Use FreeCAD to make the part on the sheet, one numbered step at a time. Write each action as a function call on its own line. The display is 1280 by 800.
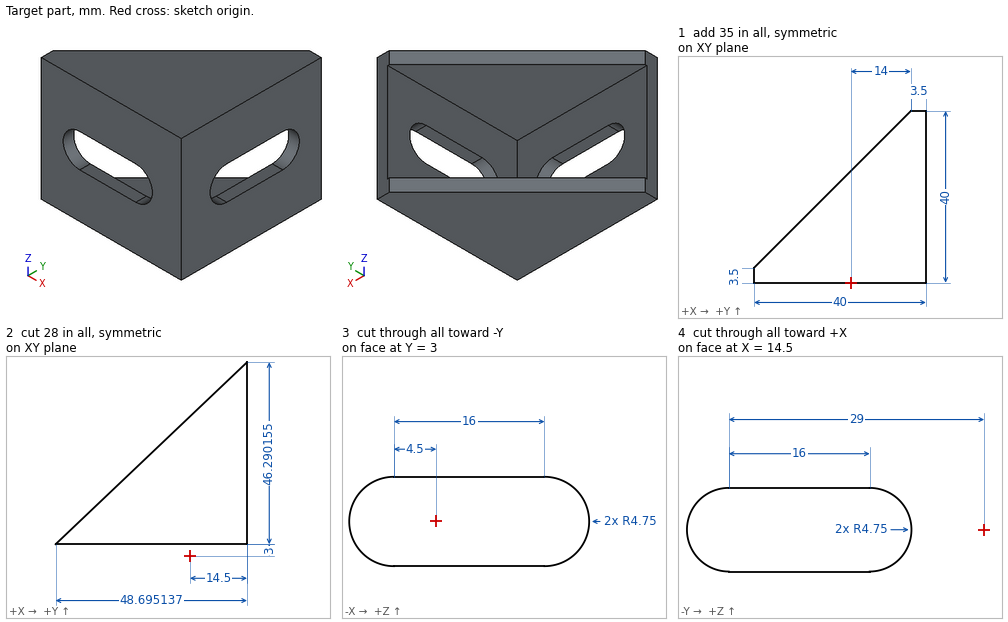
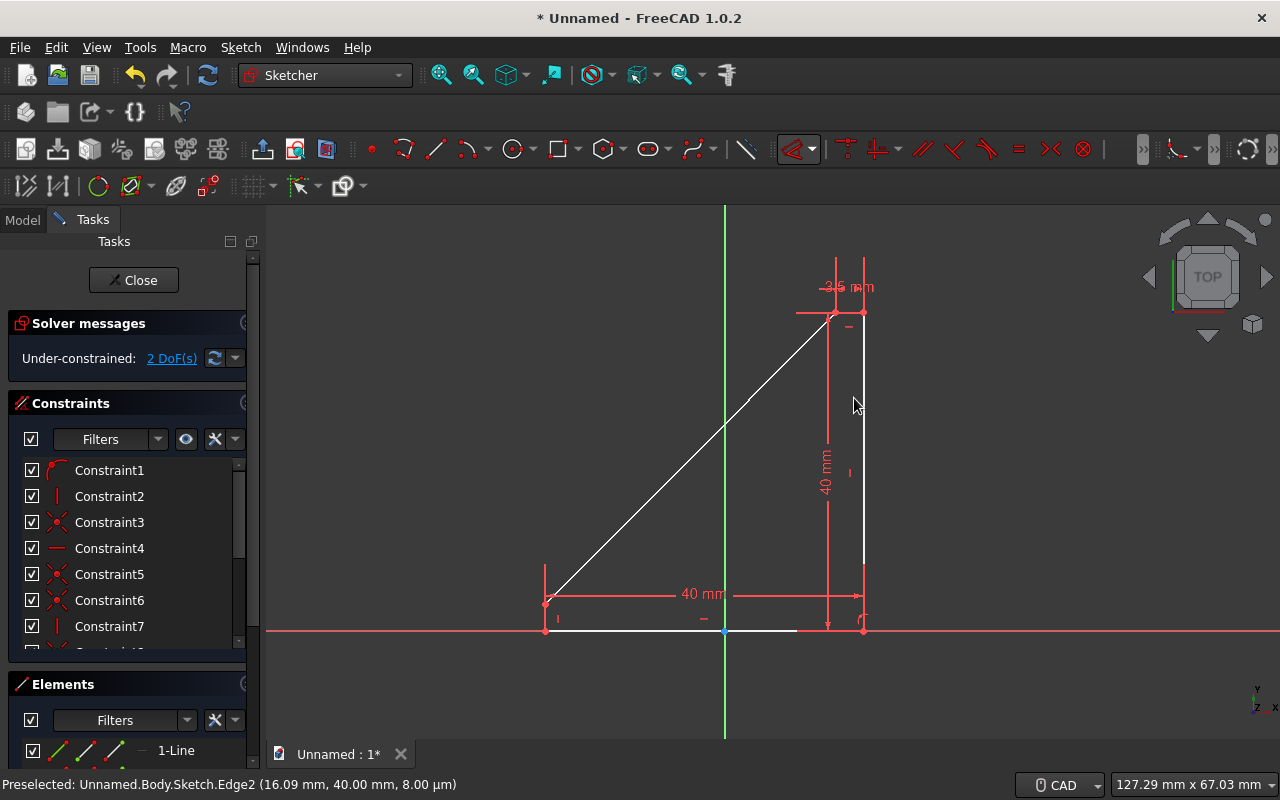
scroll(545, 613, up, 3)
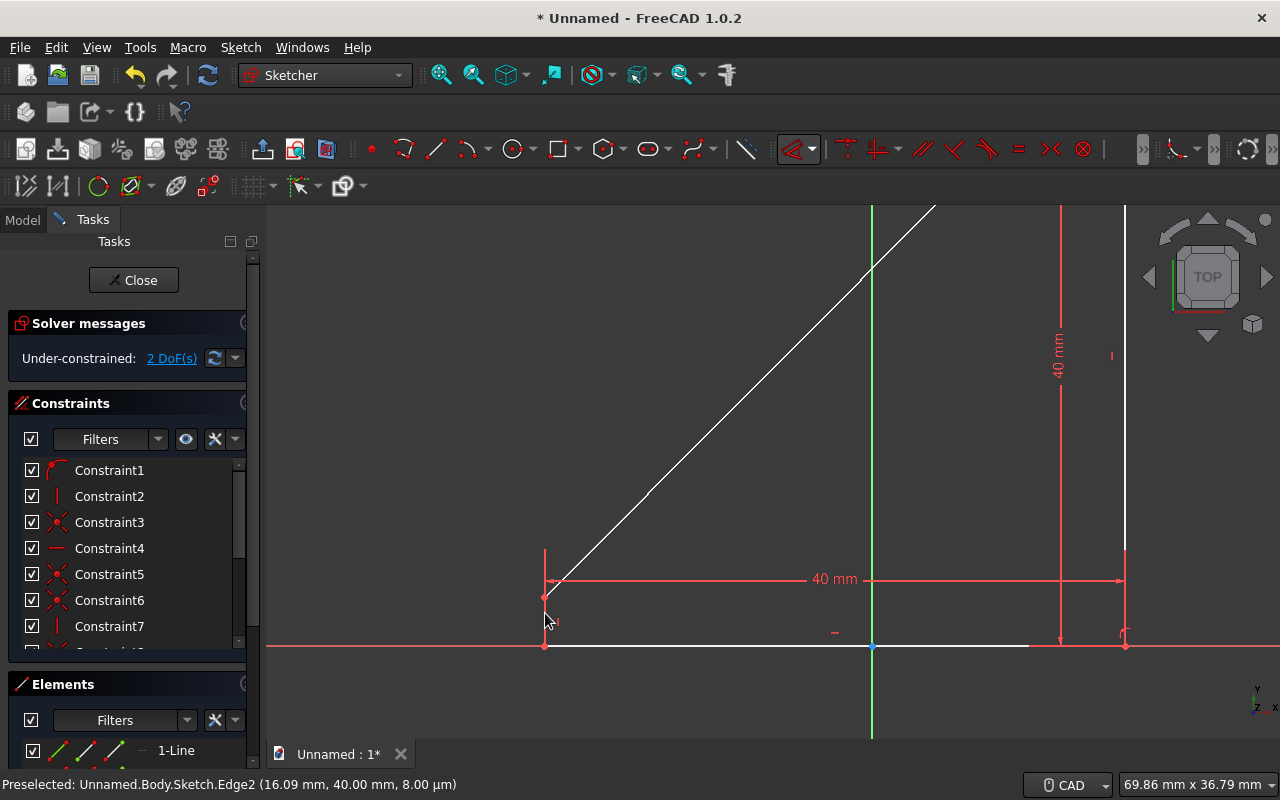
click(545, 612)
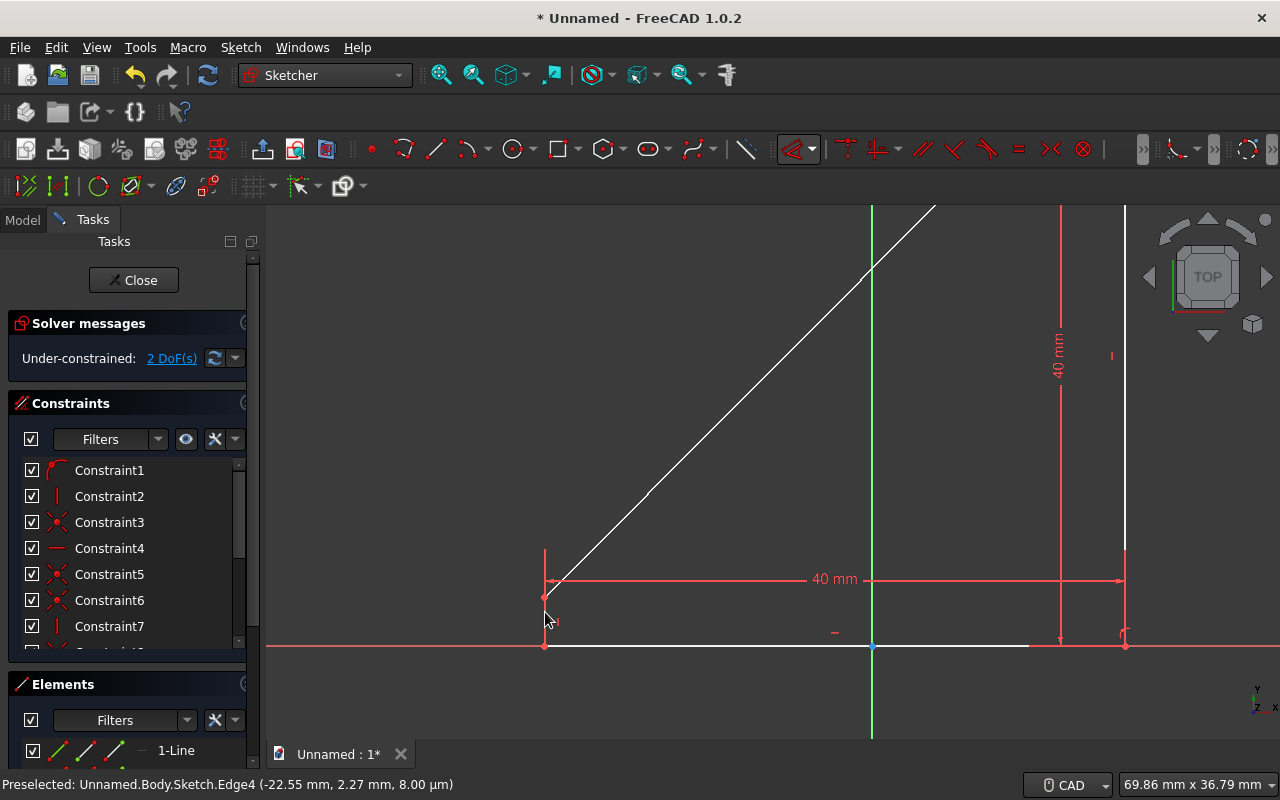
key(i)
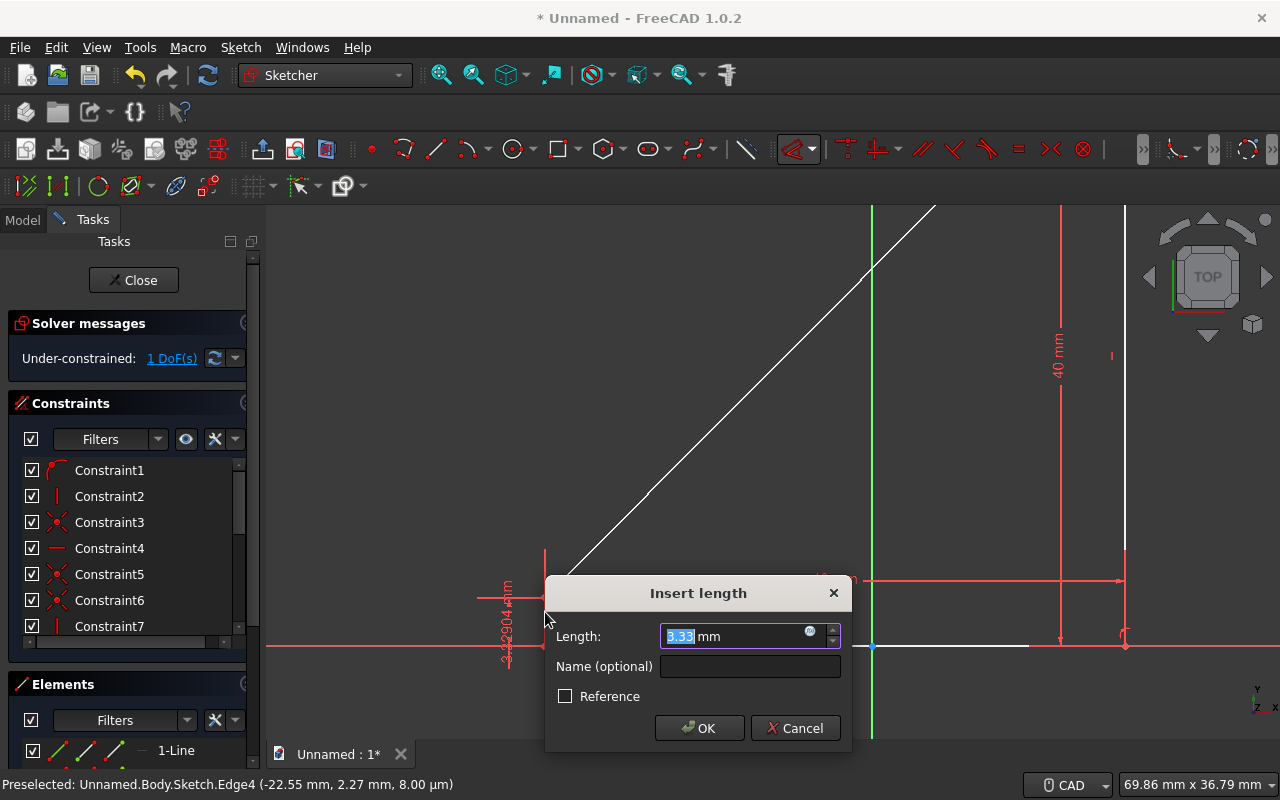
text(3.5)
key(Return)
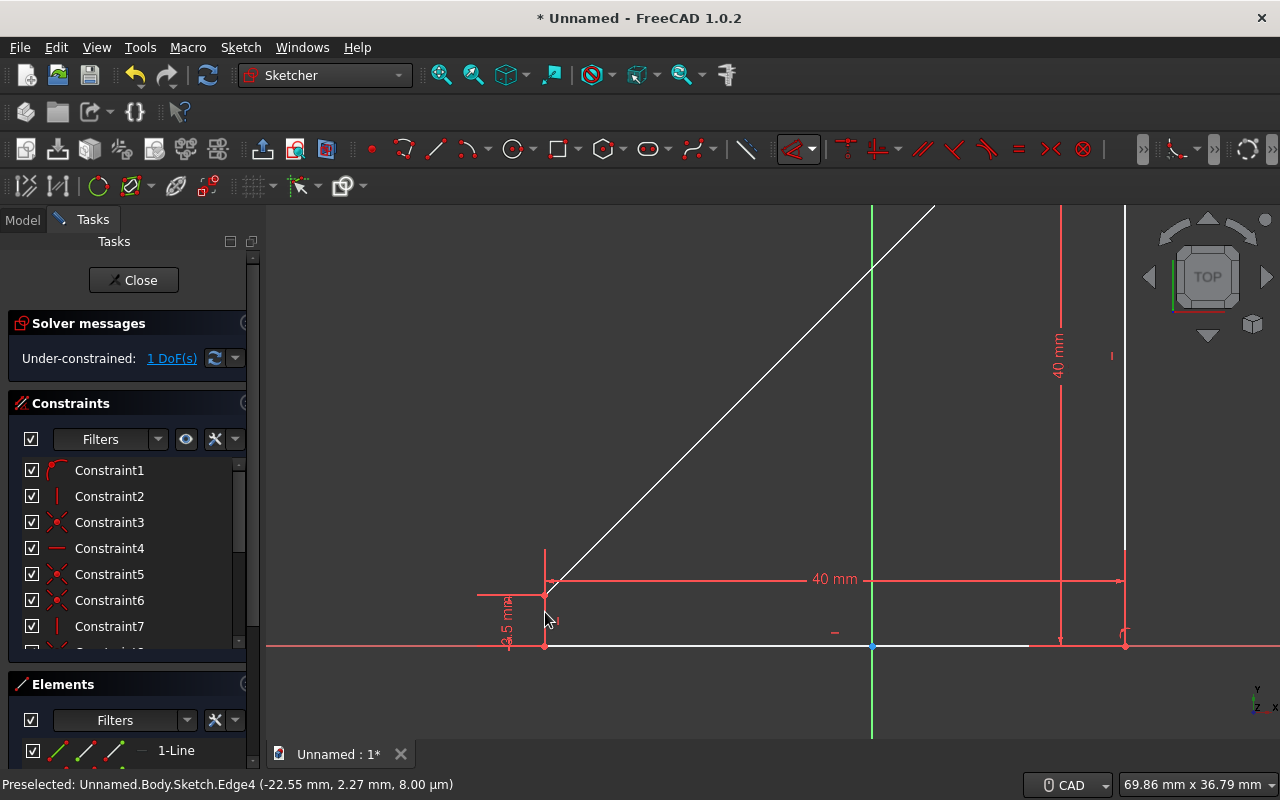
scroll(545, 613, down, 3)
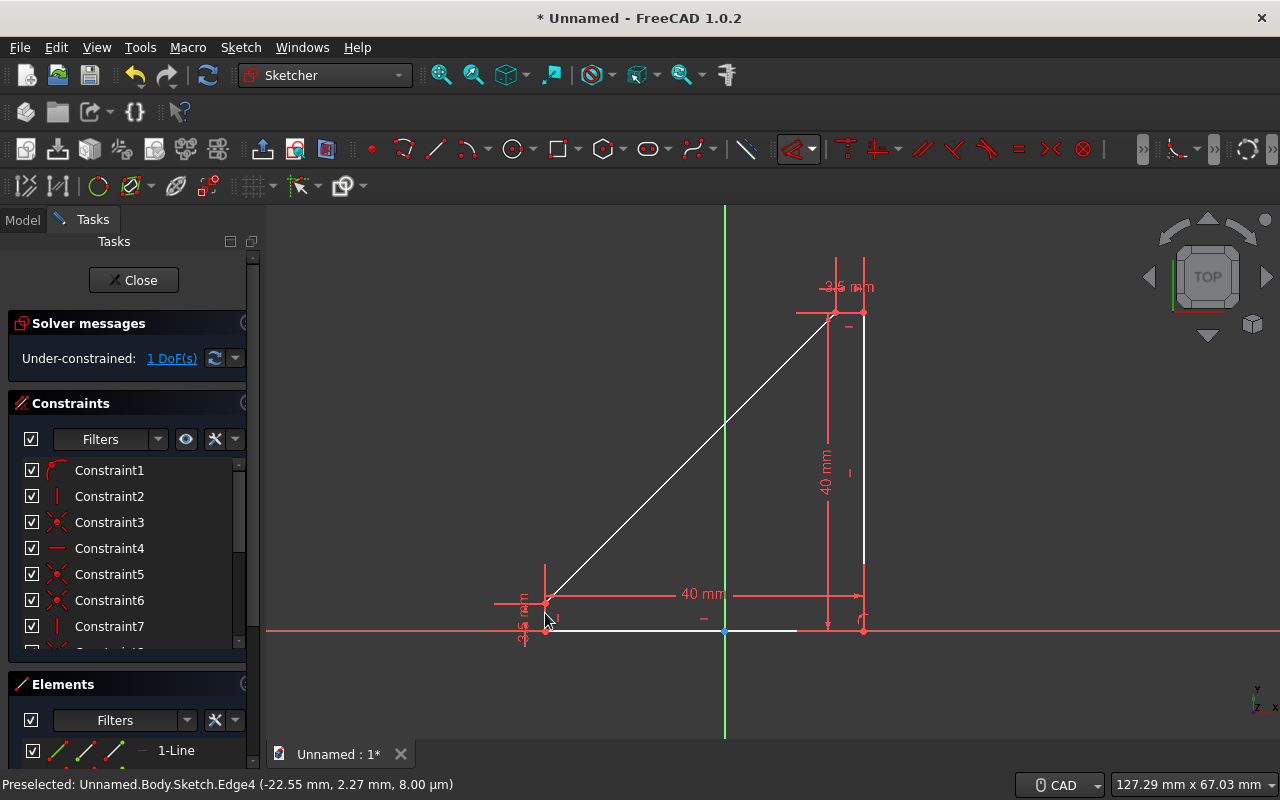
click(836, 313)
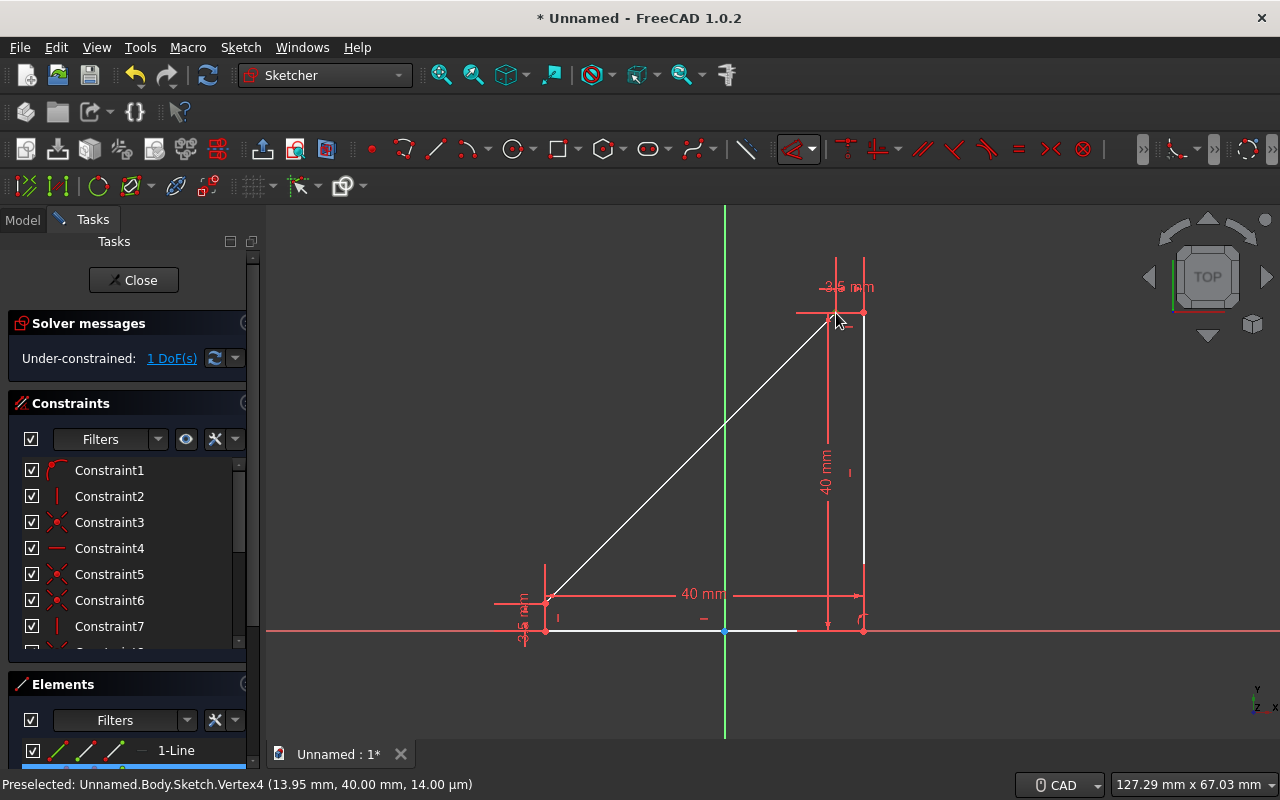
key(l)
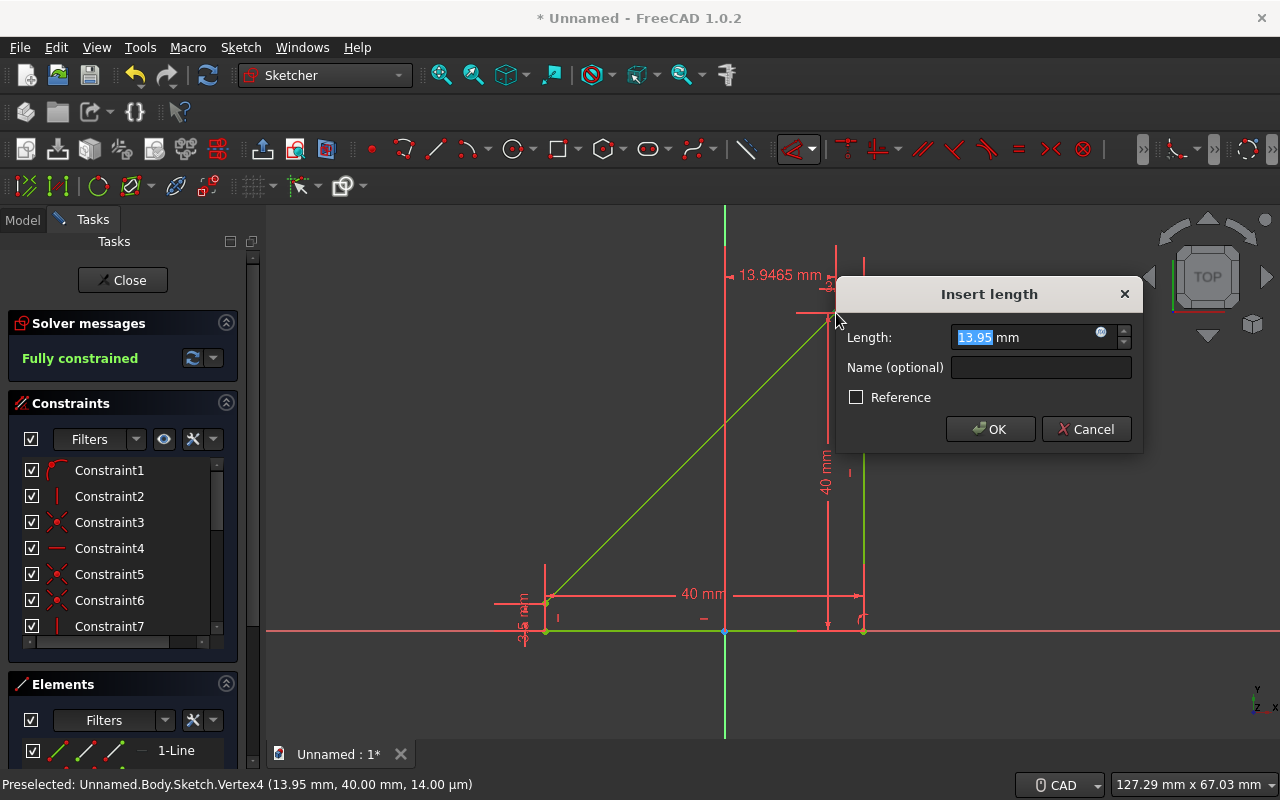
text(14)
key(Return)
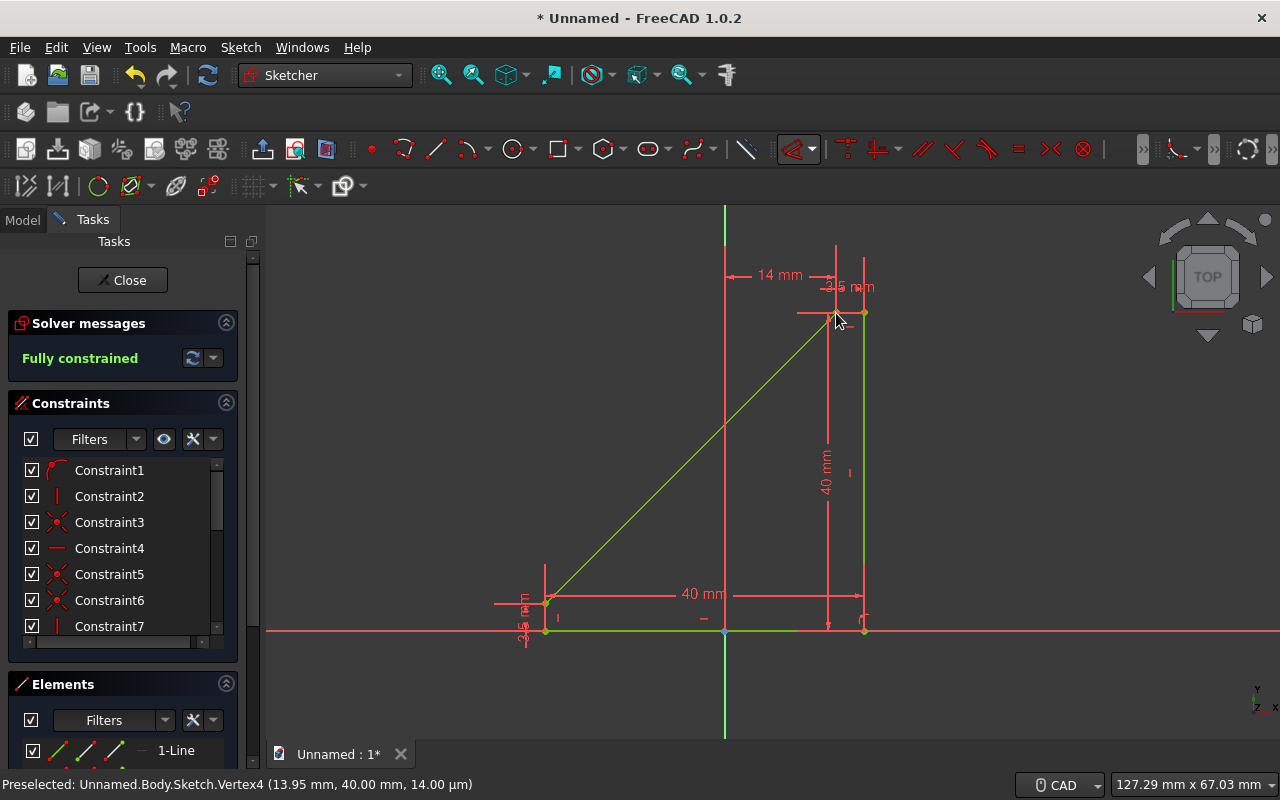
click(123, 280)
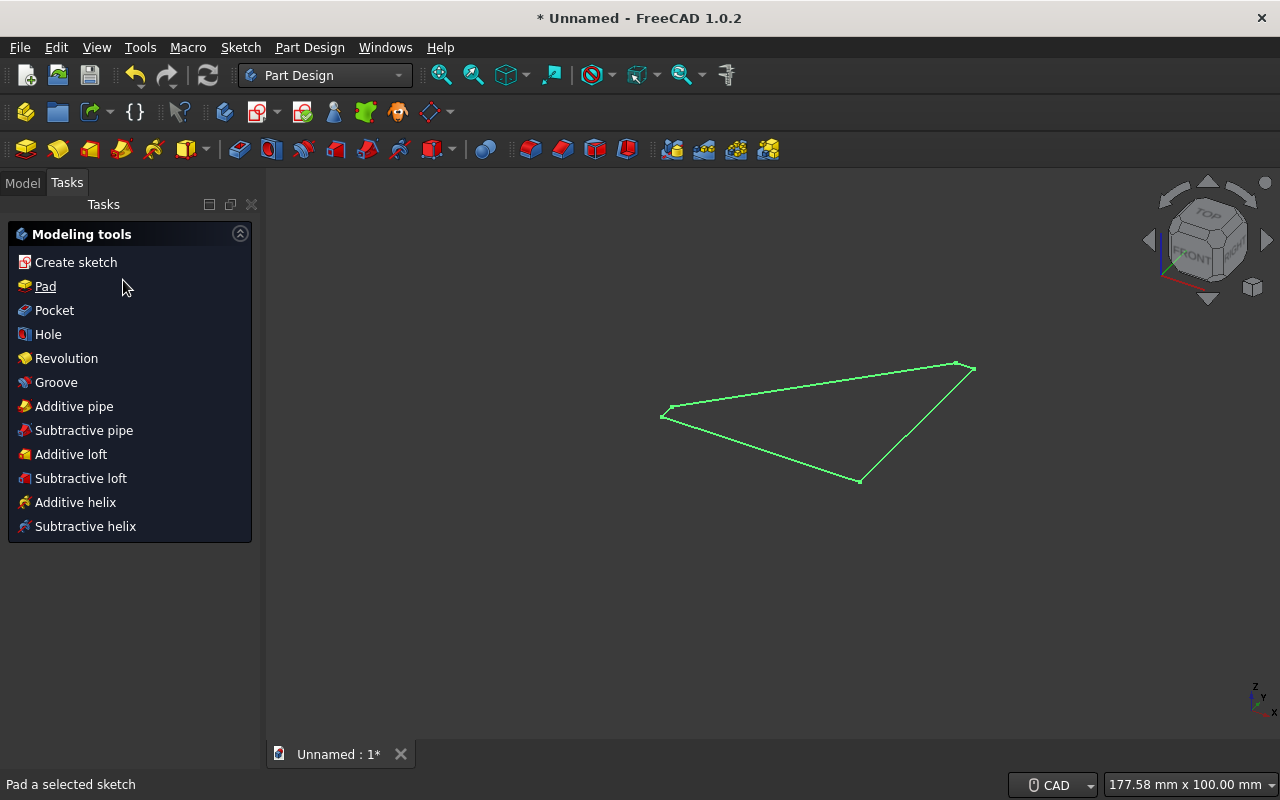
click(26, 150)